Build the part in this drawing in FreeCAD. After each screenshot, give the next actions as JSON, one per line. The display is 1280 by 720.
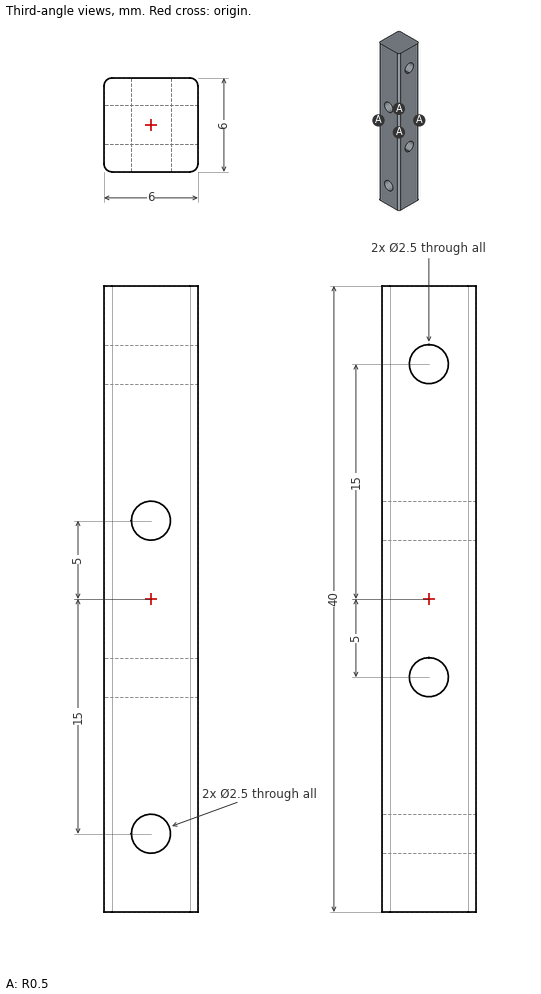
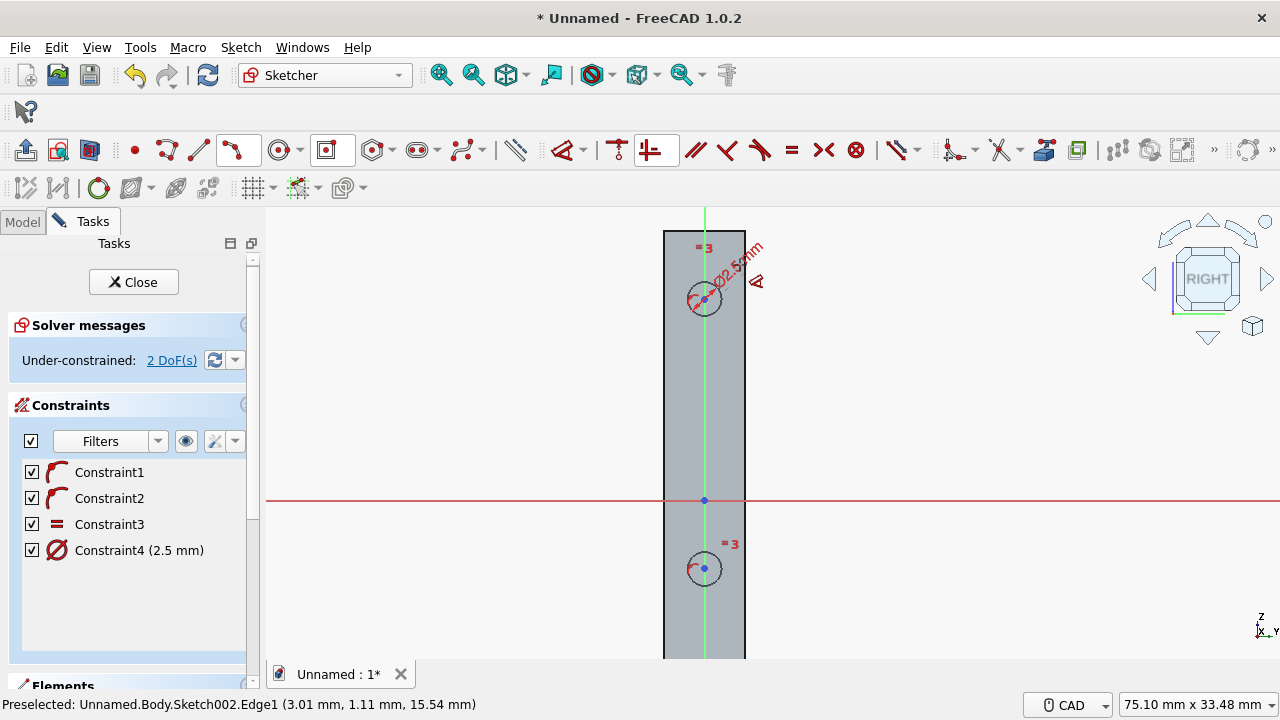
{"action": "left_click", "coordinate": [705, 569]}
{"action": "left_click", "coordinate": [739, 535]}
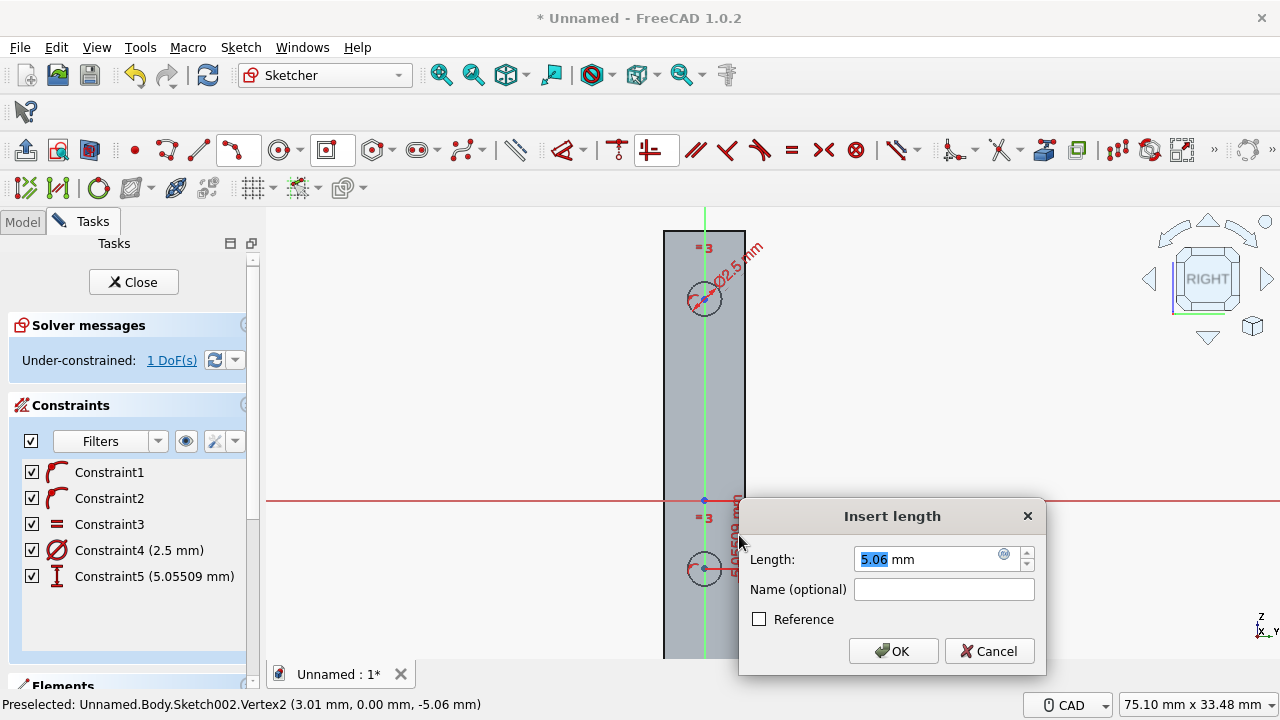
{"action": "type", "text": "5"}
{"action": "key", "text": "Return"}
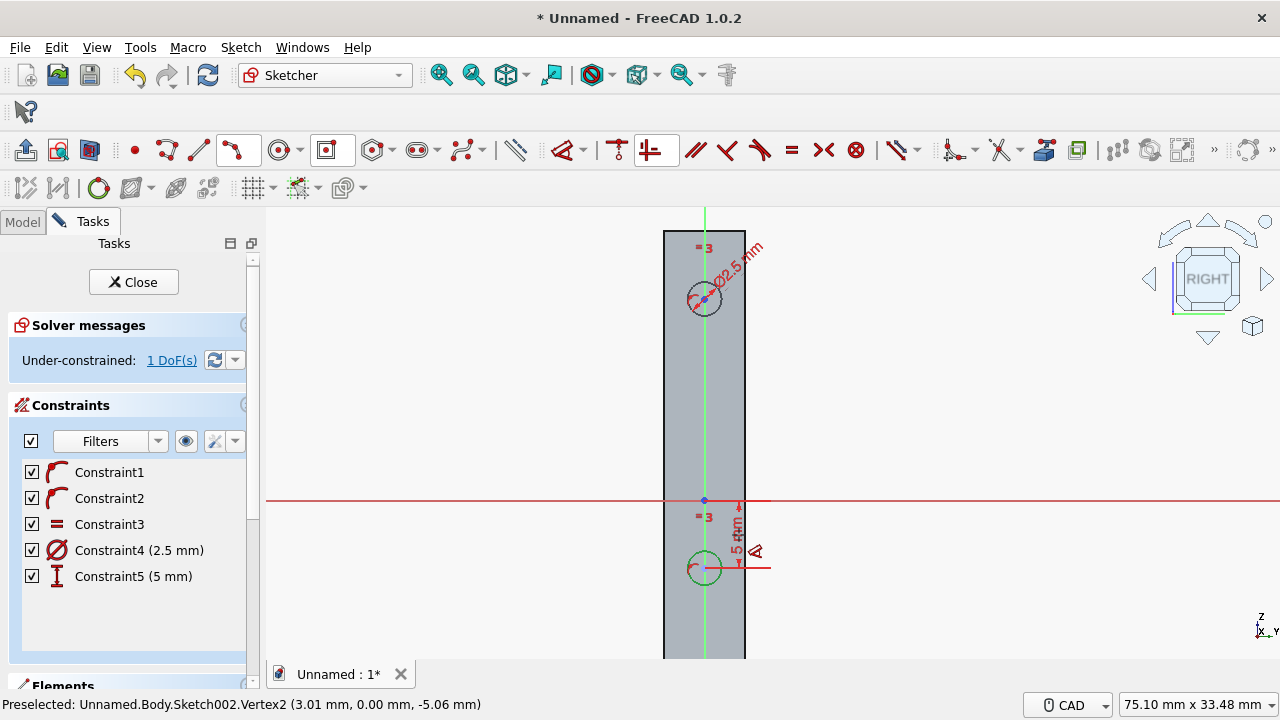
{"action": "left_click", "coordinate": [705, 299]}
{"action": "left_click", "coordinate": [739, 400]}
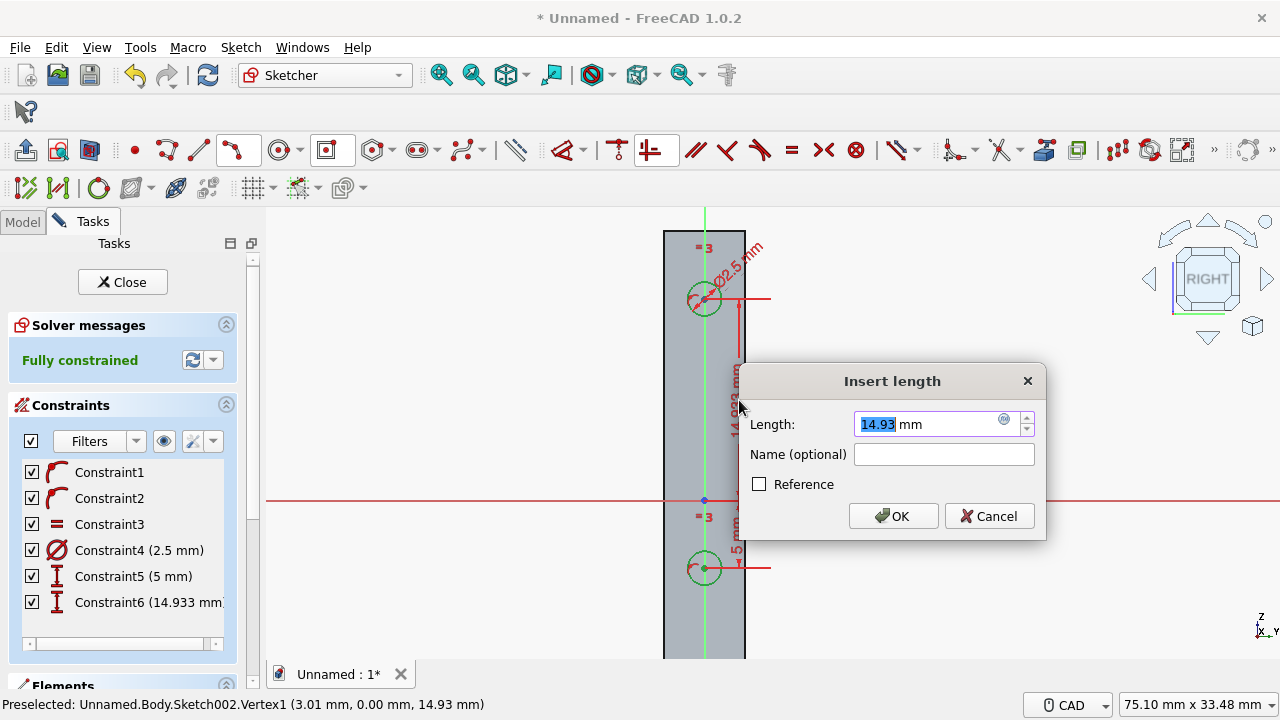
{"action": "type", "text": "15"}
{"action": "key", "text": "Return"}
{"action": "key", "text": "Escape"}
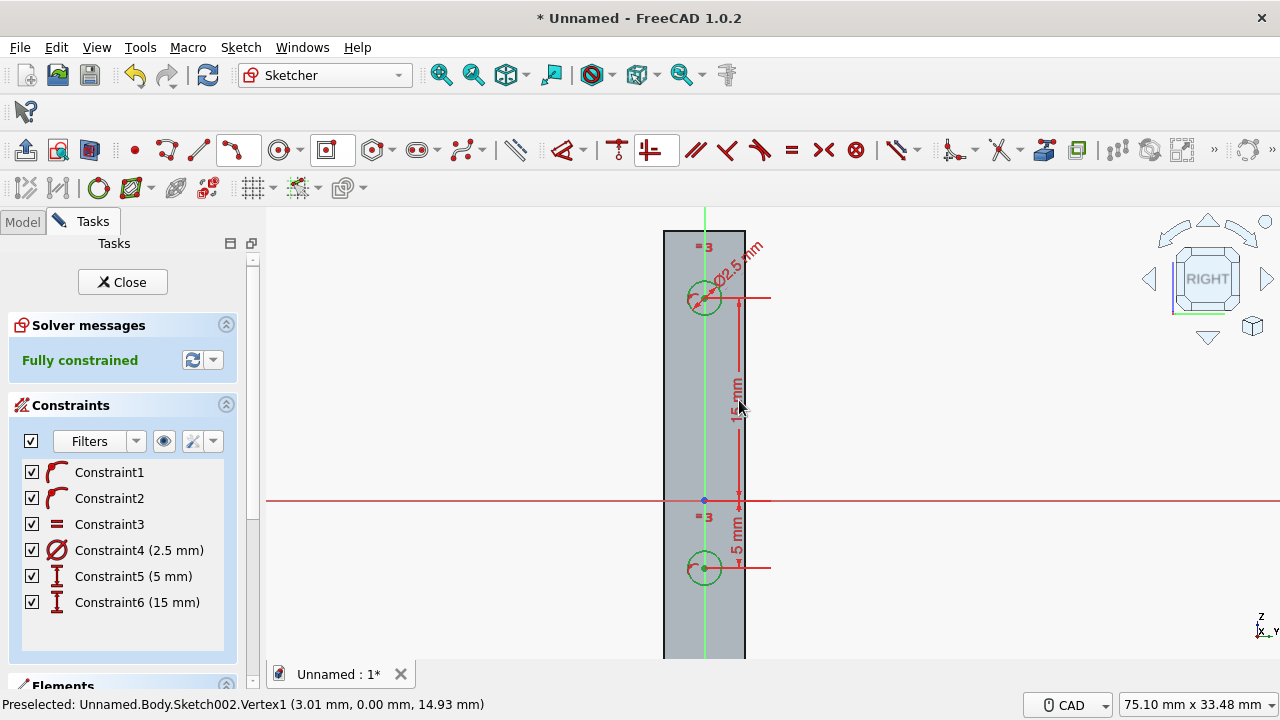
{"action": "left_click", "coordinate": [123, 282]}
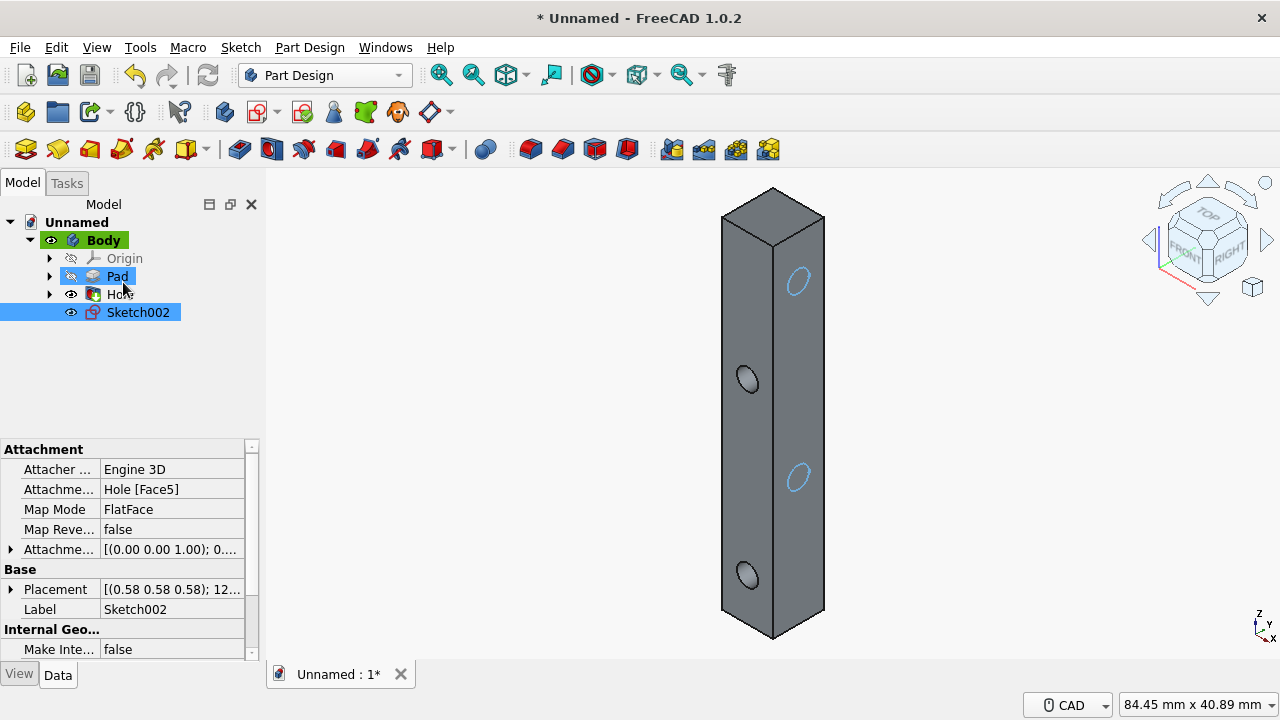
{"action": "left_click", "coordinate": [272, 150]}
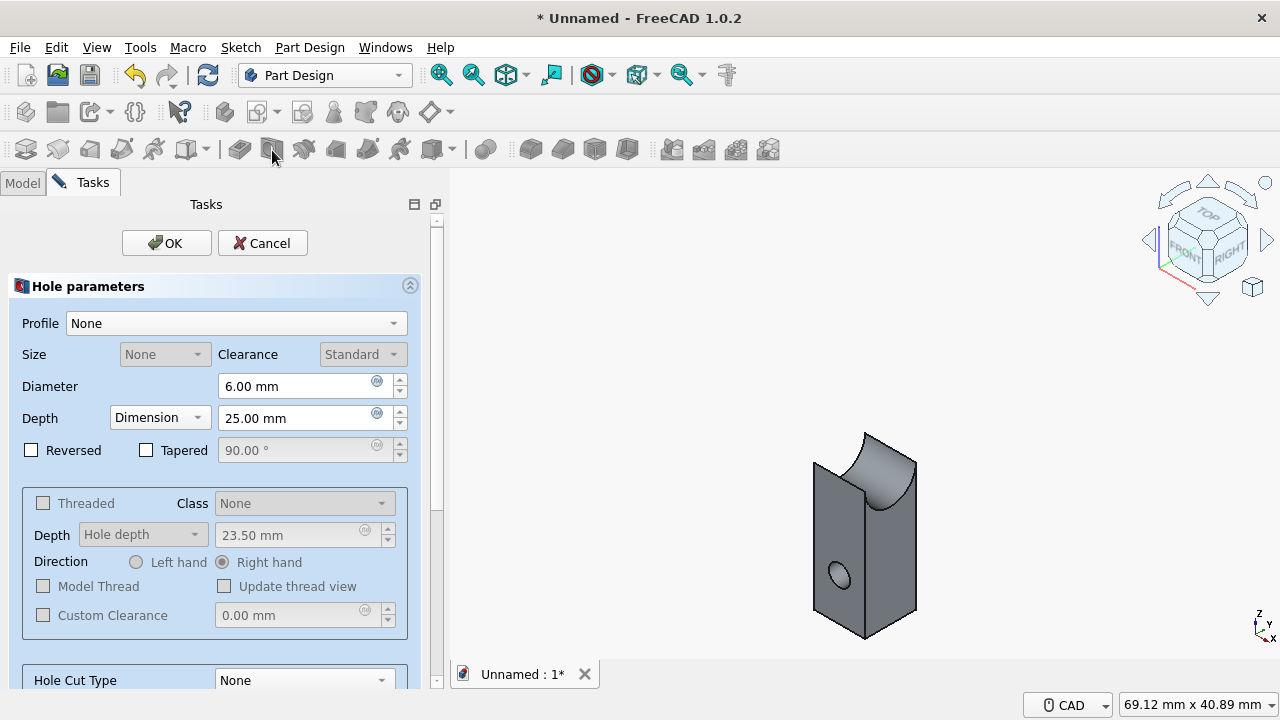
{"action": "triple_click", "coordinate": [305, 386]}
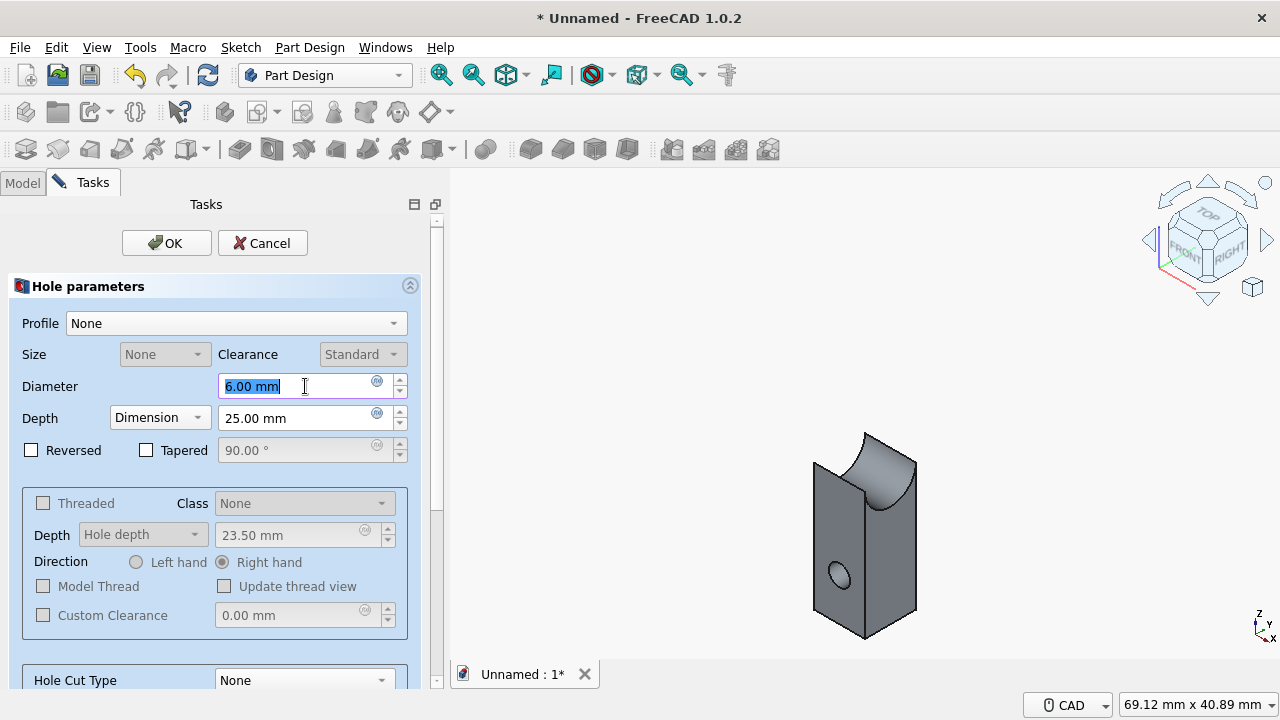
{"action": "type", "text": "2.5"}
{"action": "key", "text": "Tab"}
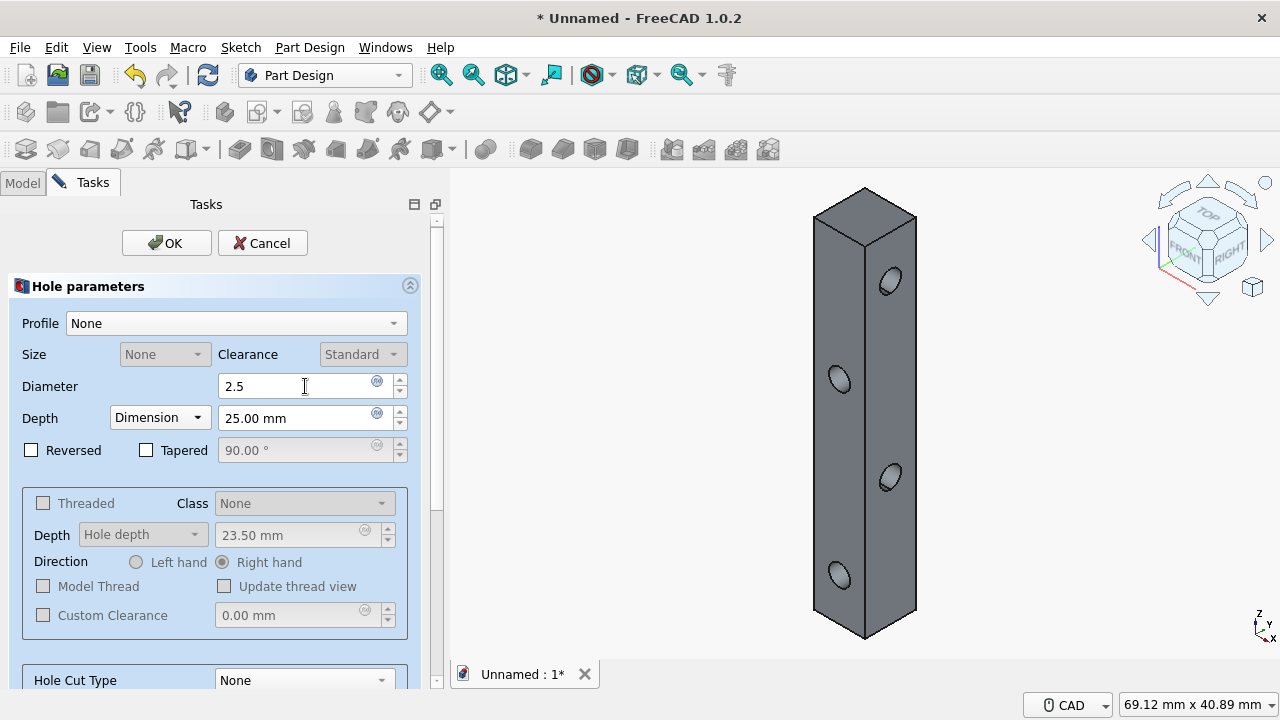
{"action": "left_click", "coordinate": [161, 418]}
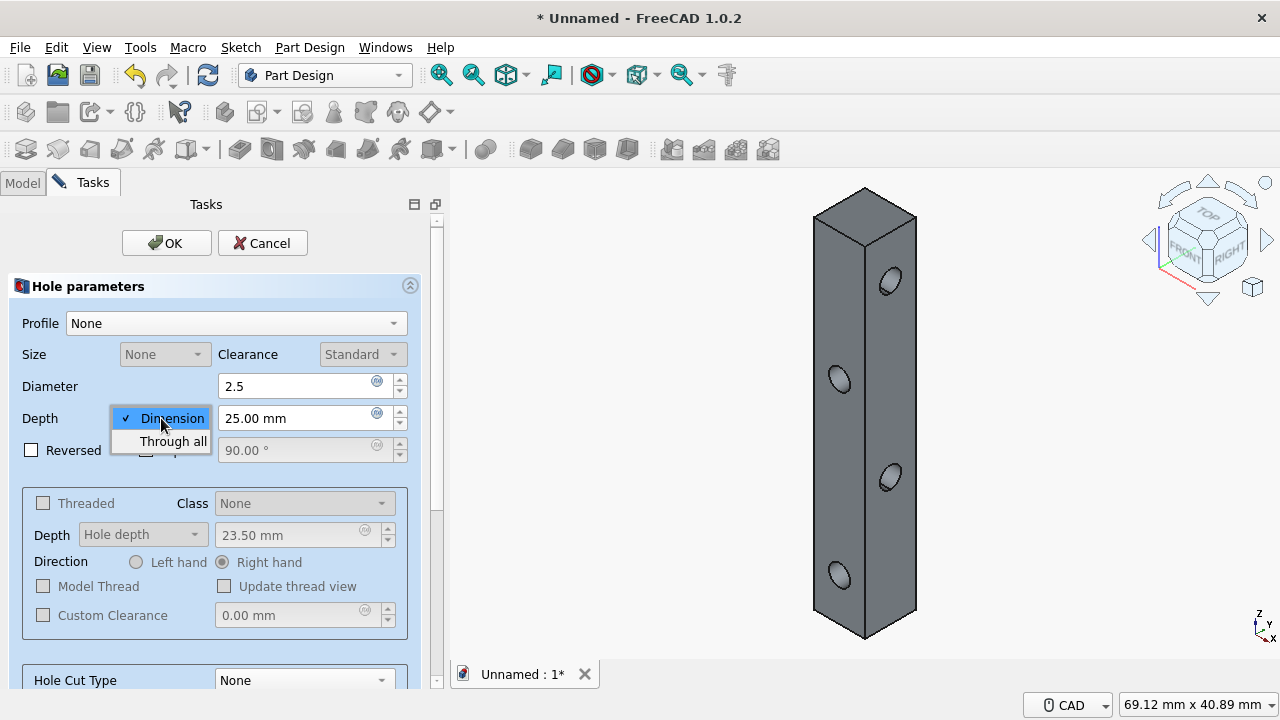
{"action": "left_click", "coordinate": [160, 442]}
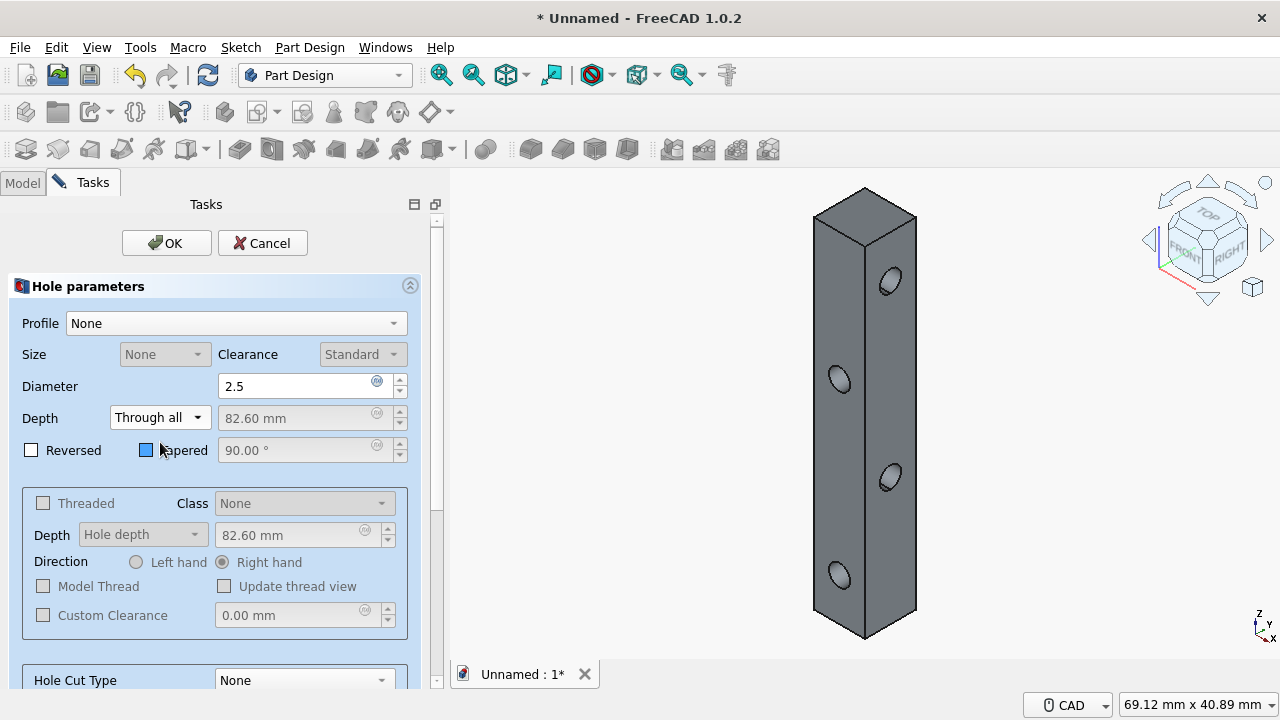
{"action": "left_click", "coordinate": [167, 243]}